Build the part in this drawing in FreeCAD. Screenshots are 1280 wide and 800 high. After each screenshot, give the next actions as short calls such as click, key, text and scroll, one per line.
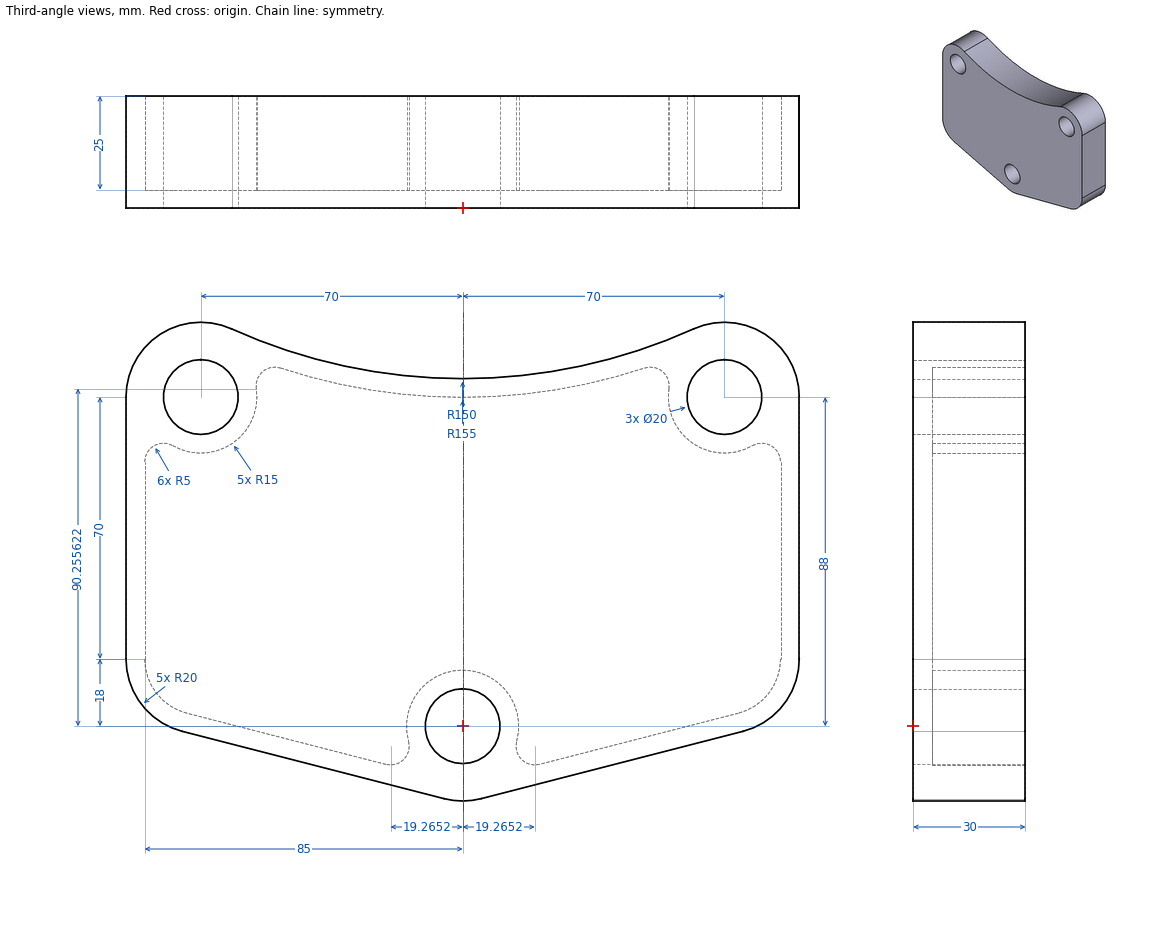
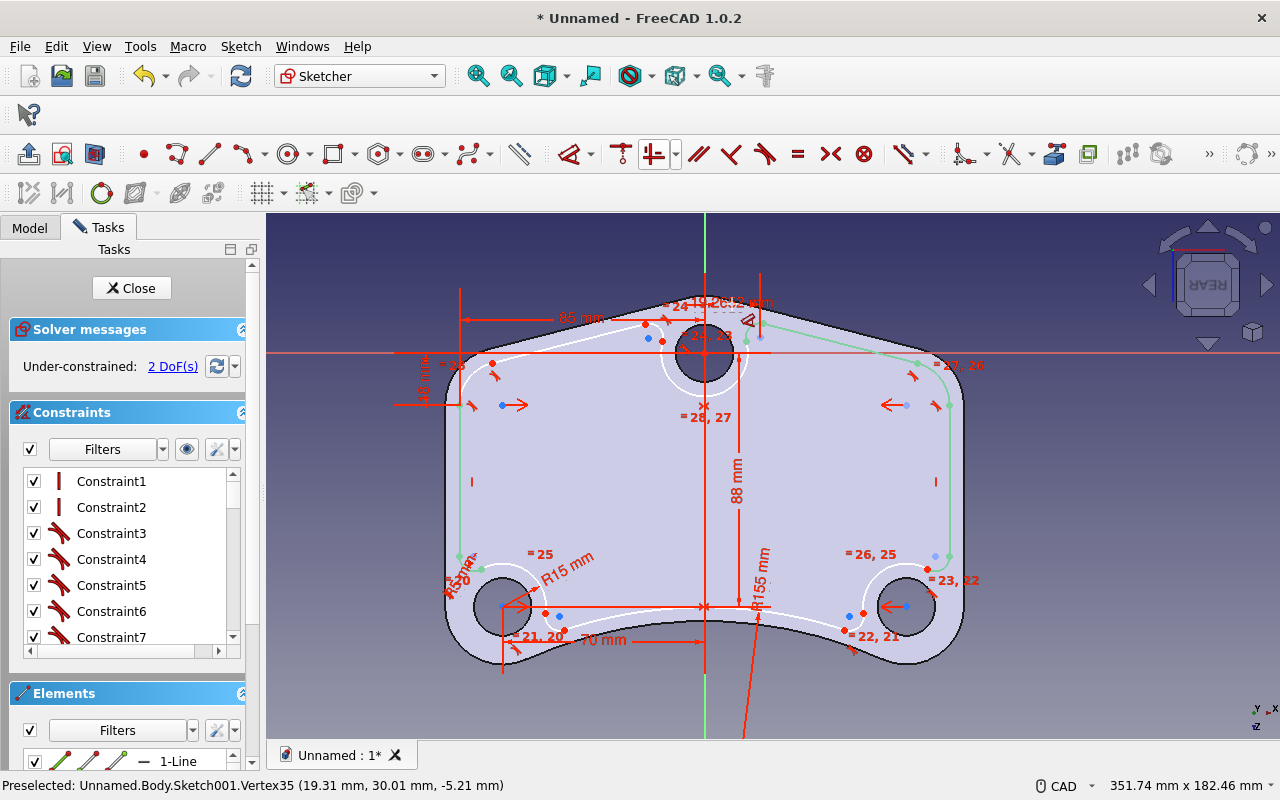
click(649, 338)
click(657, 304)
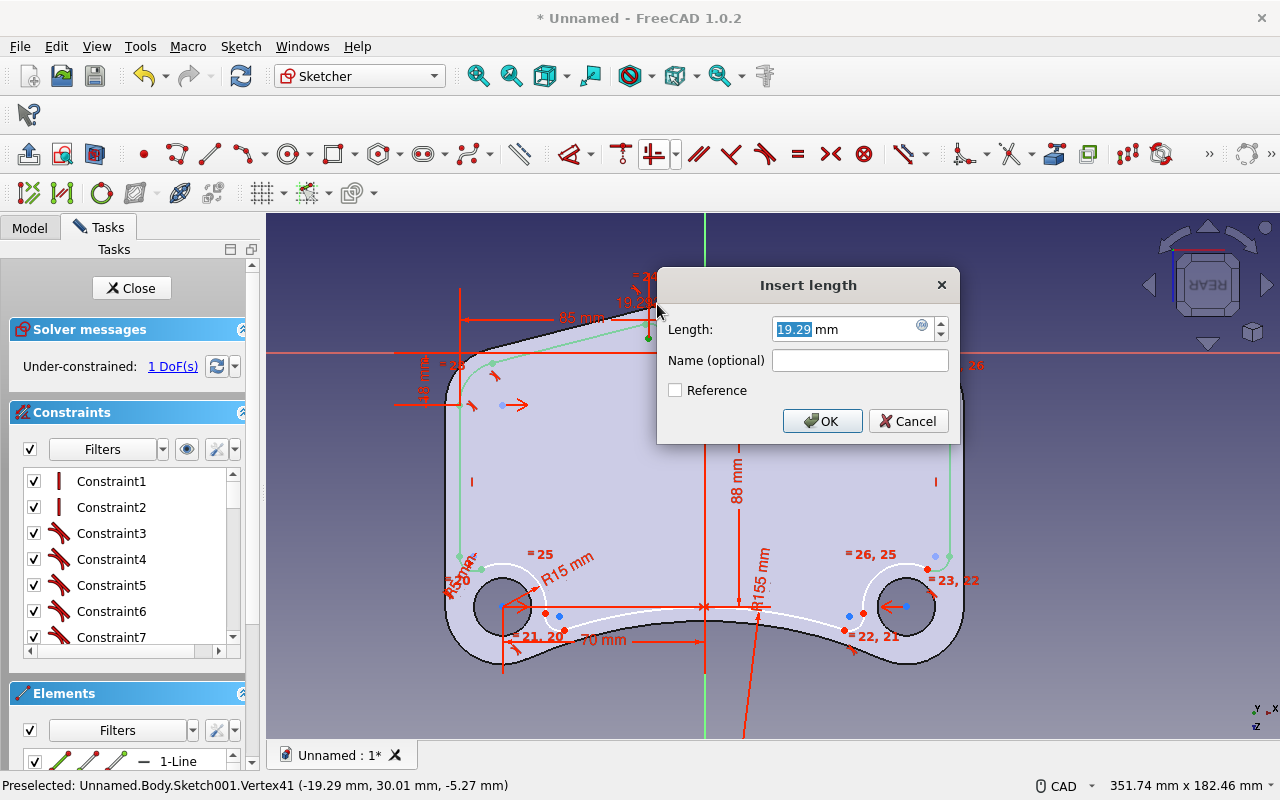
text(19.2652)
key(Return)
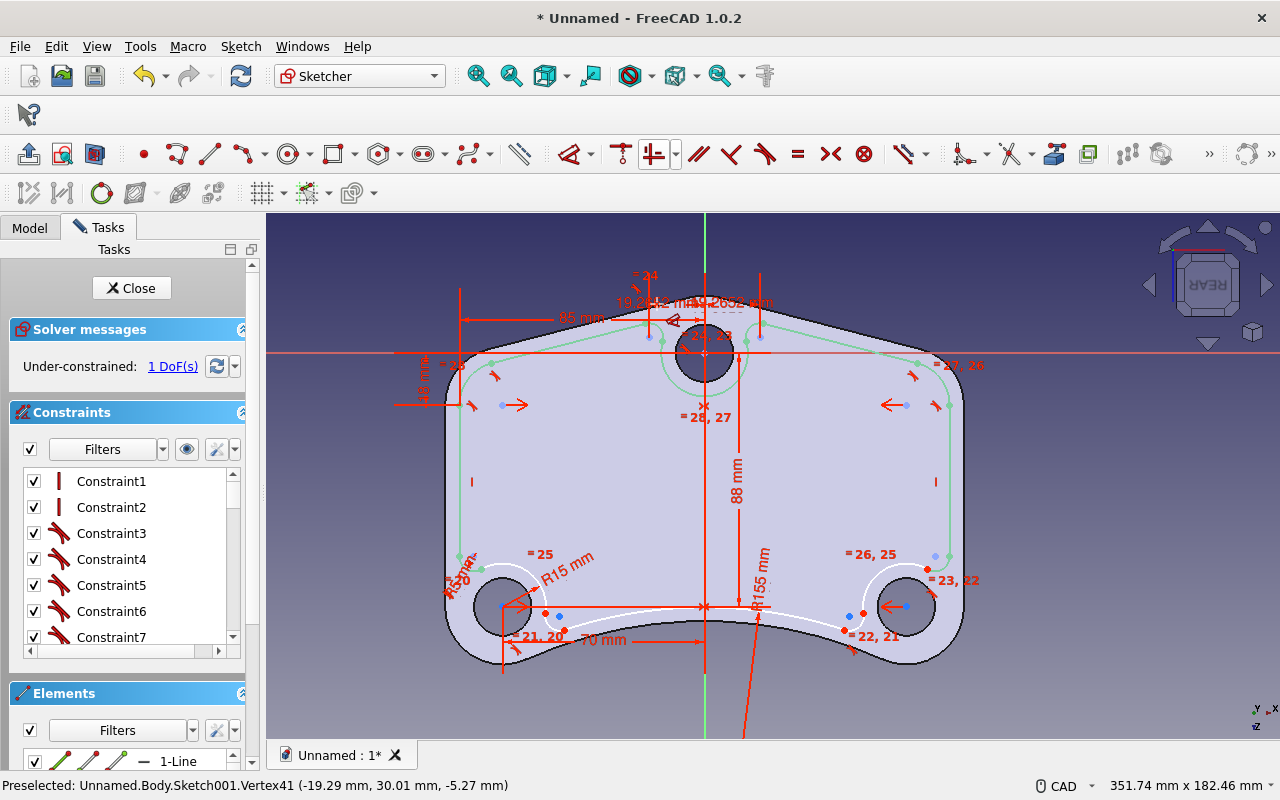
click(545, 614)
click(511, 484)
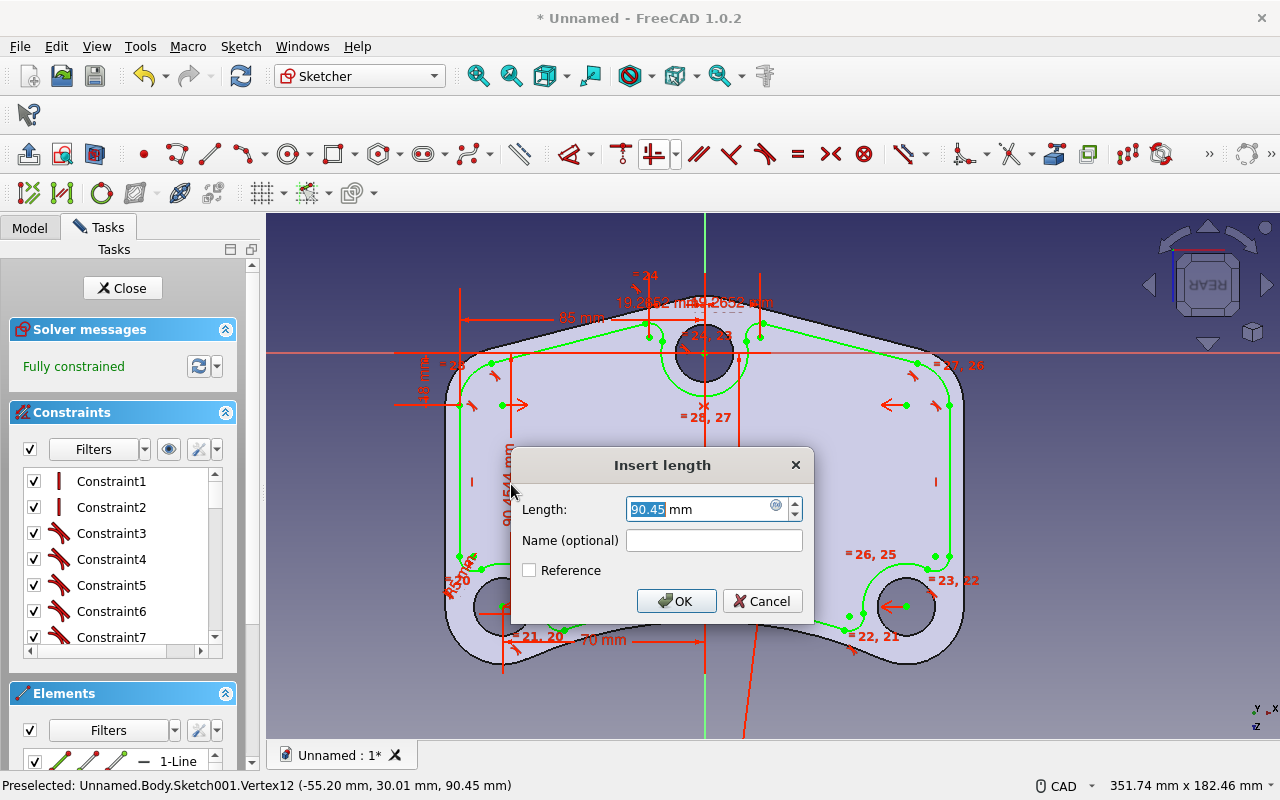
text(90.255622)
key(Return)
key(Escape)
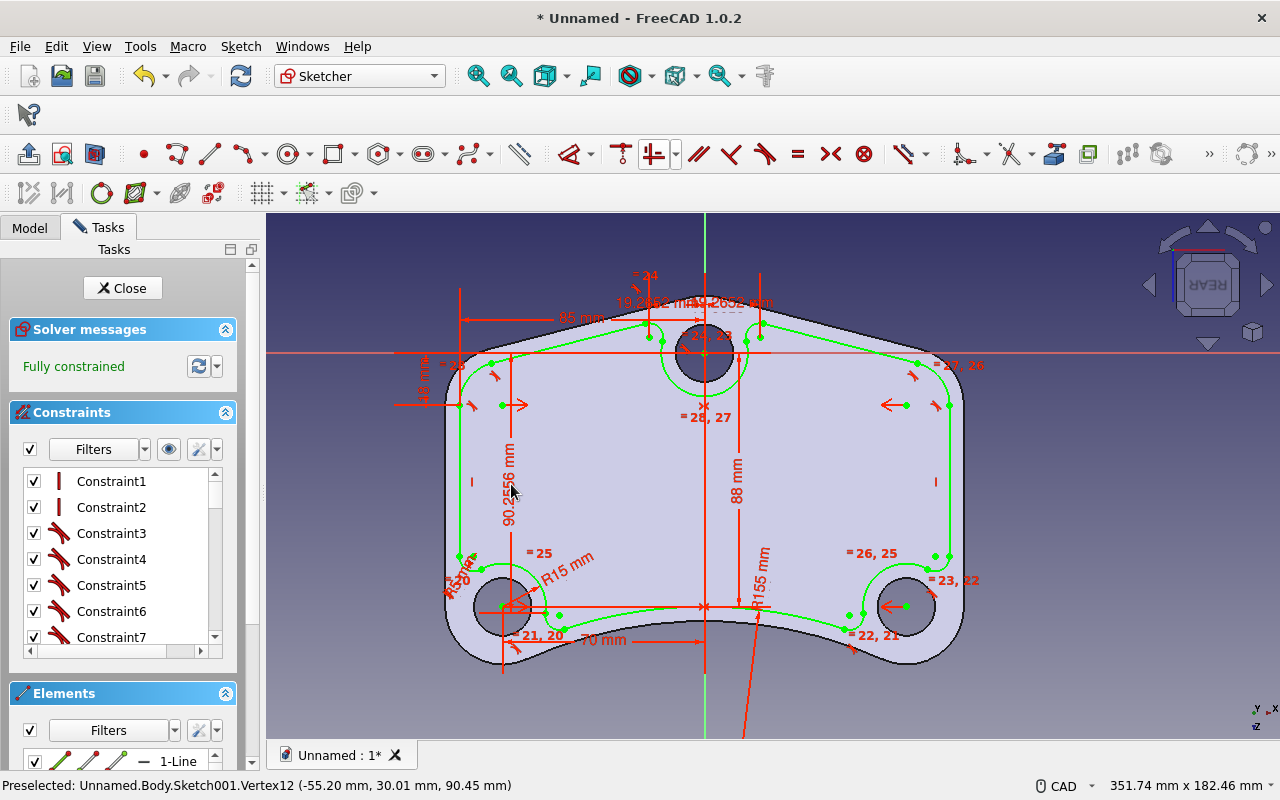
click(123, 288)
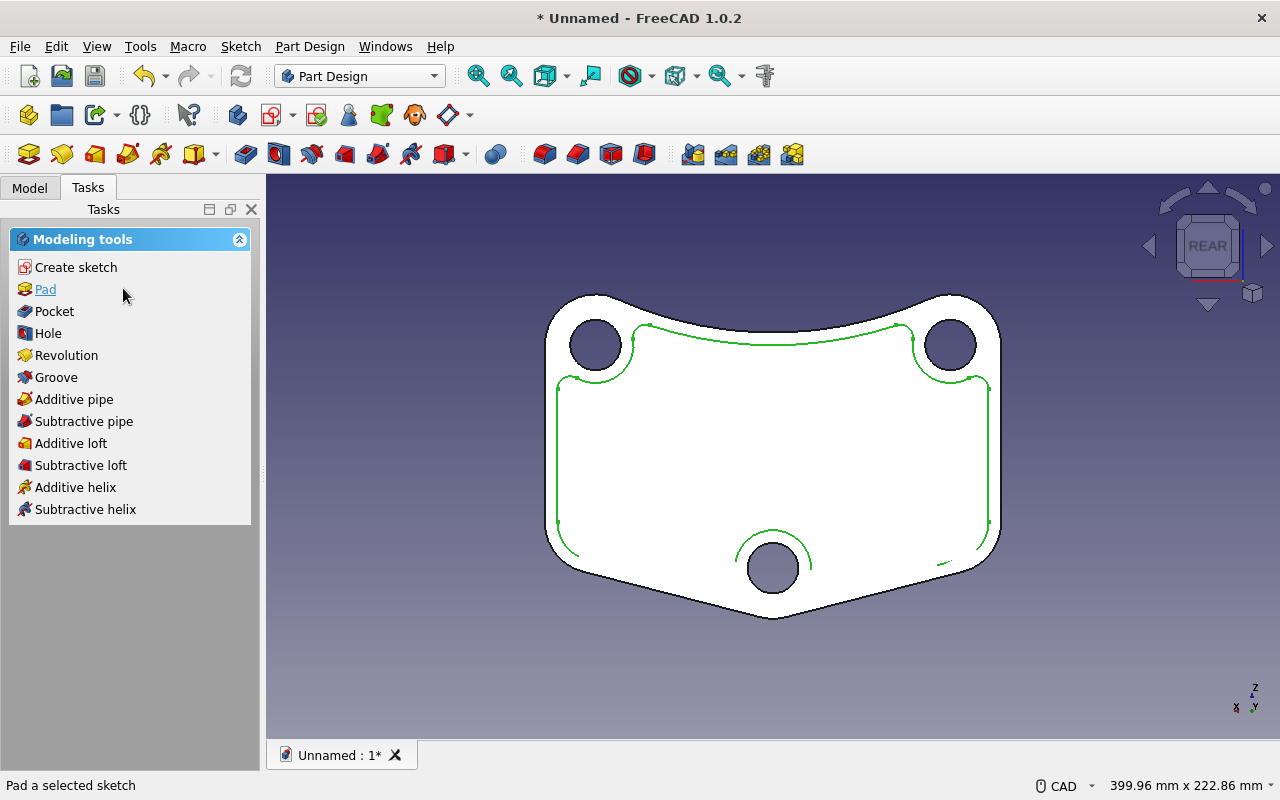
click(246, 154)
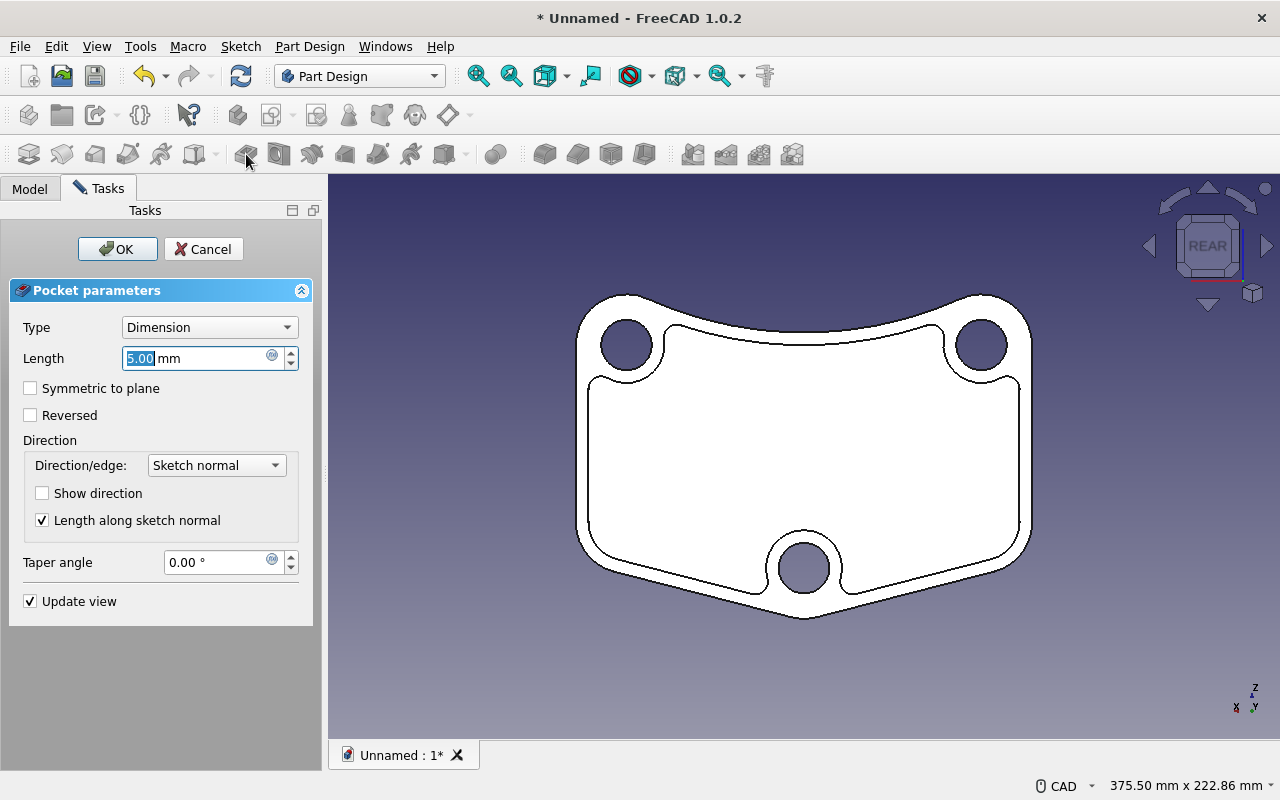
text(25)
key(Tab)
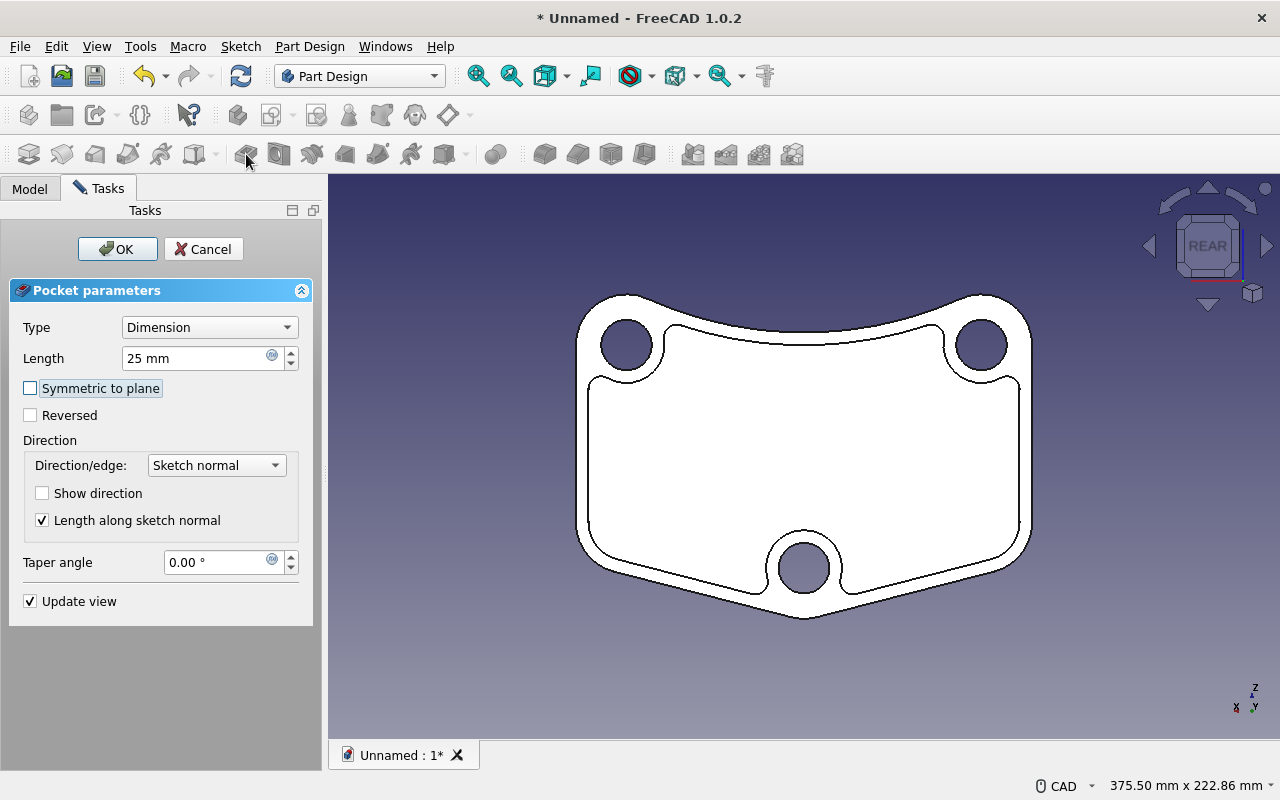
click(118, 249)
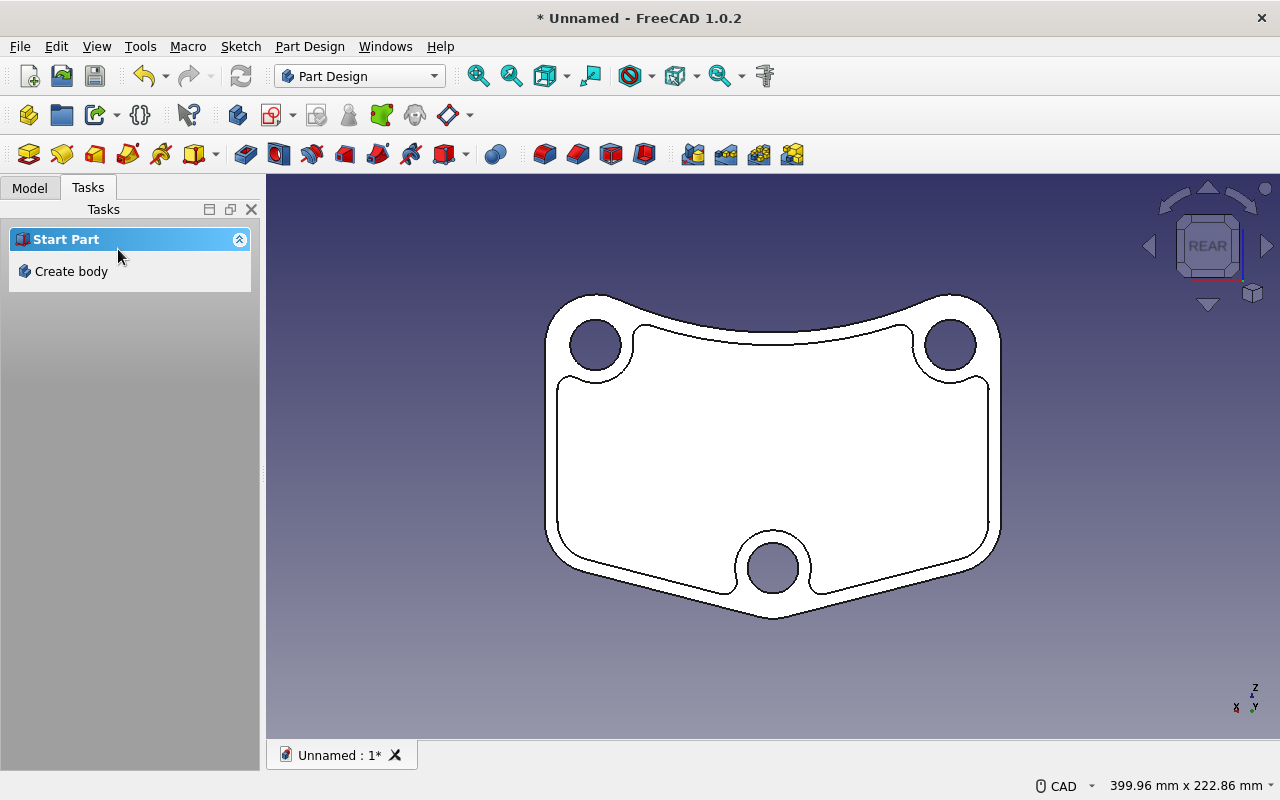
key(0)